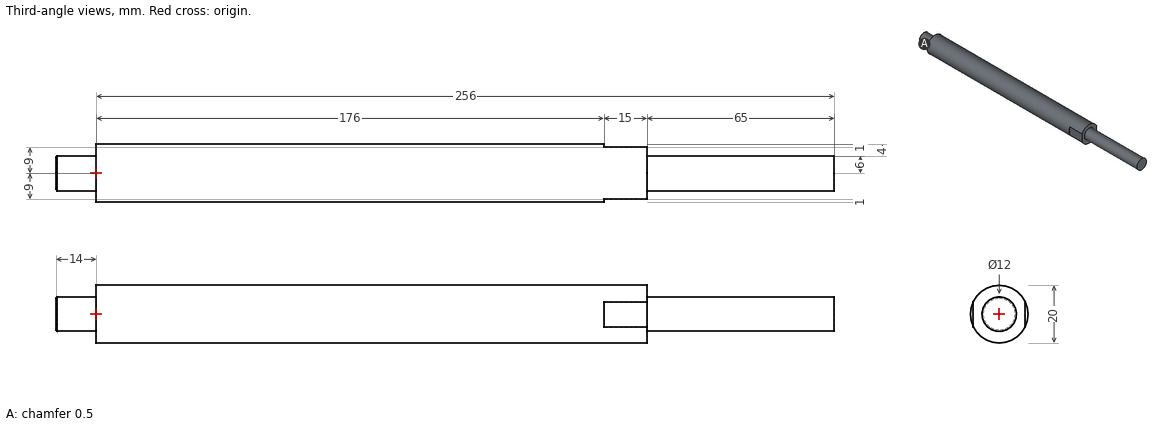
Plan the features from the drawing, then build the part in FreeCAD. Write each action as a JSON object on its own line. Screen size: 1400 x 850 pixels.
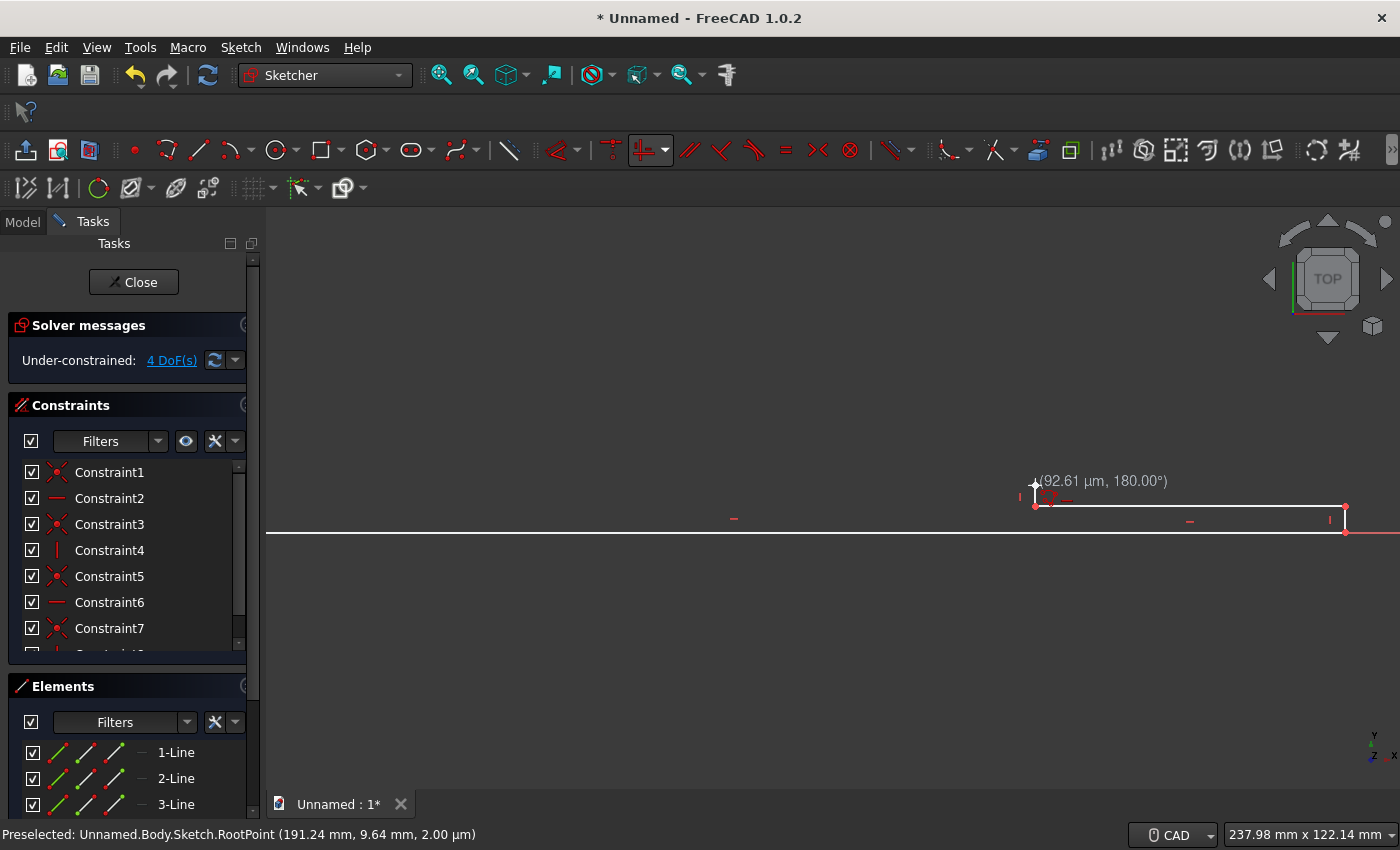
{"action": "scroll", "coordinate": [801, 485], "scroll_direction": "down", "scroll_amount": 3}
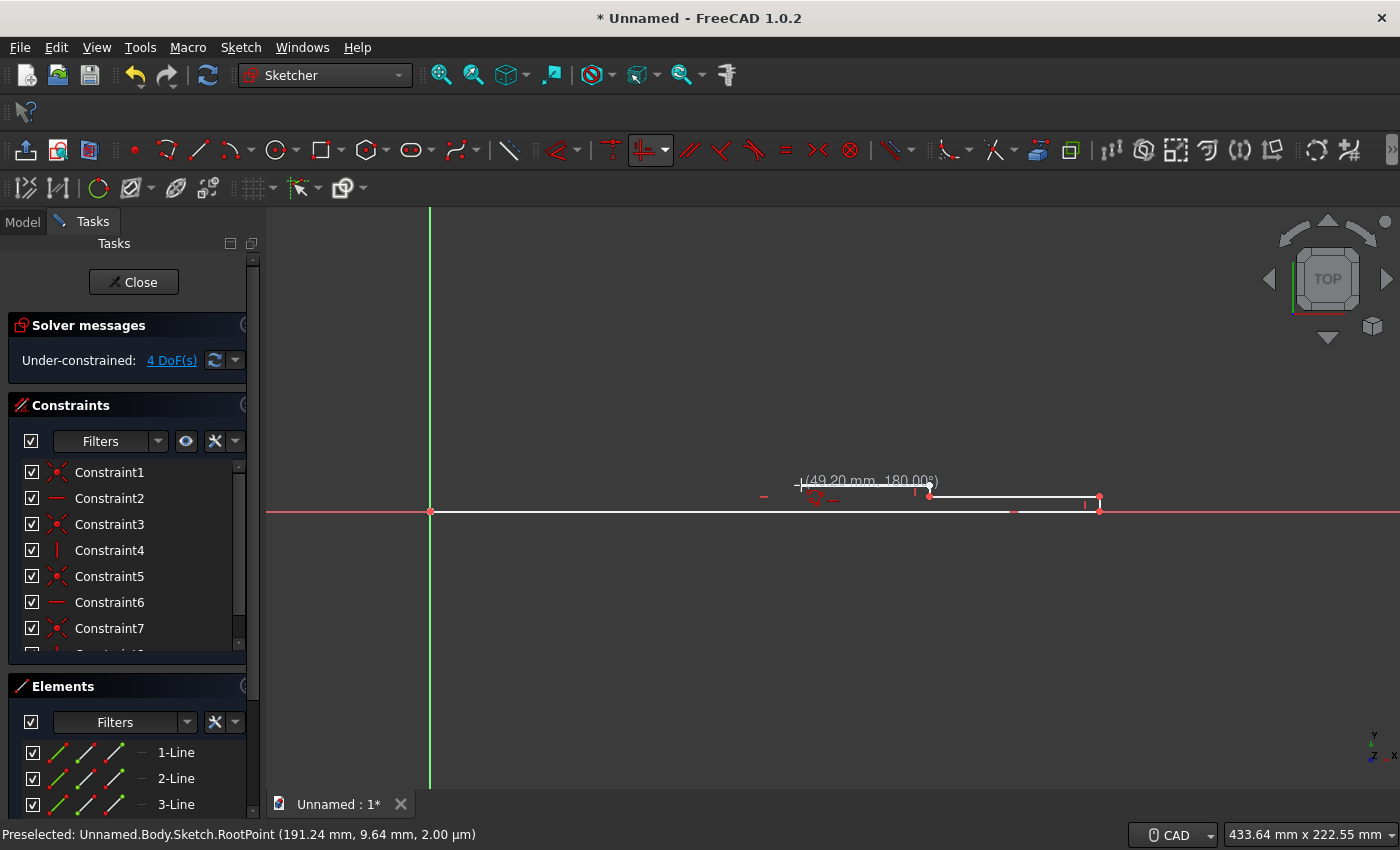
{"action": "left_click", "coordinate": [439, 485]}
{"action": "left_click", "coordinate": [430, 512]}
{"action": "key", "text": "Escape"}
{"action": "key", "text": "Escape"}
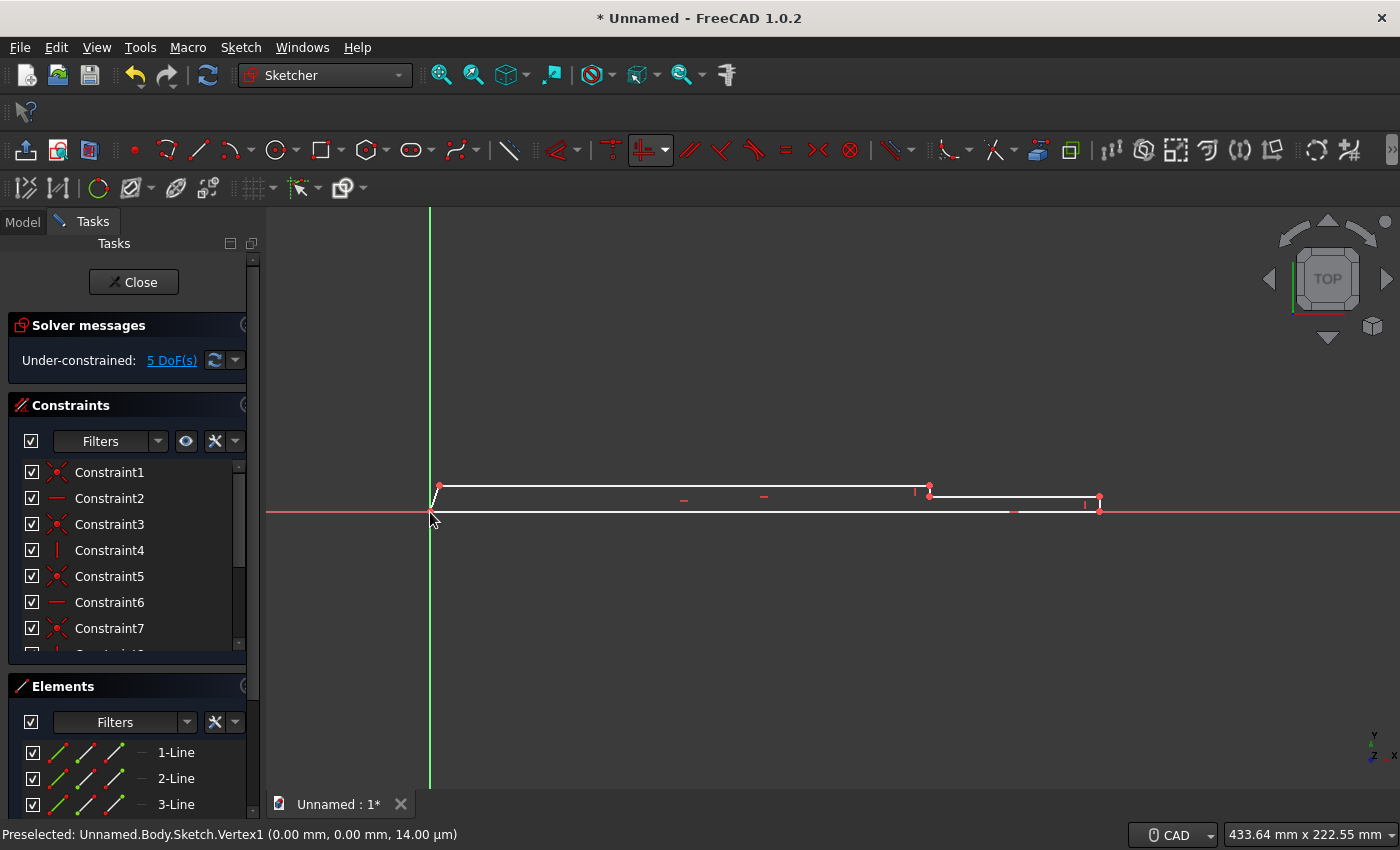
{"action": "scroll", "coordinate": [434, 501], "scroll_direction": "up", "scroll_amount": 2}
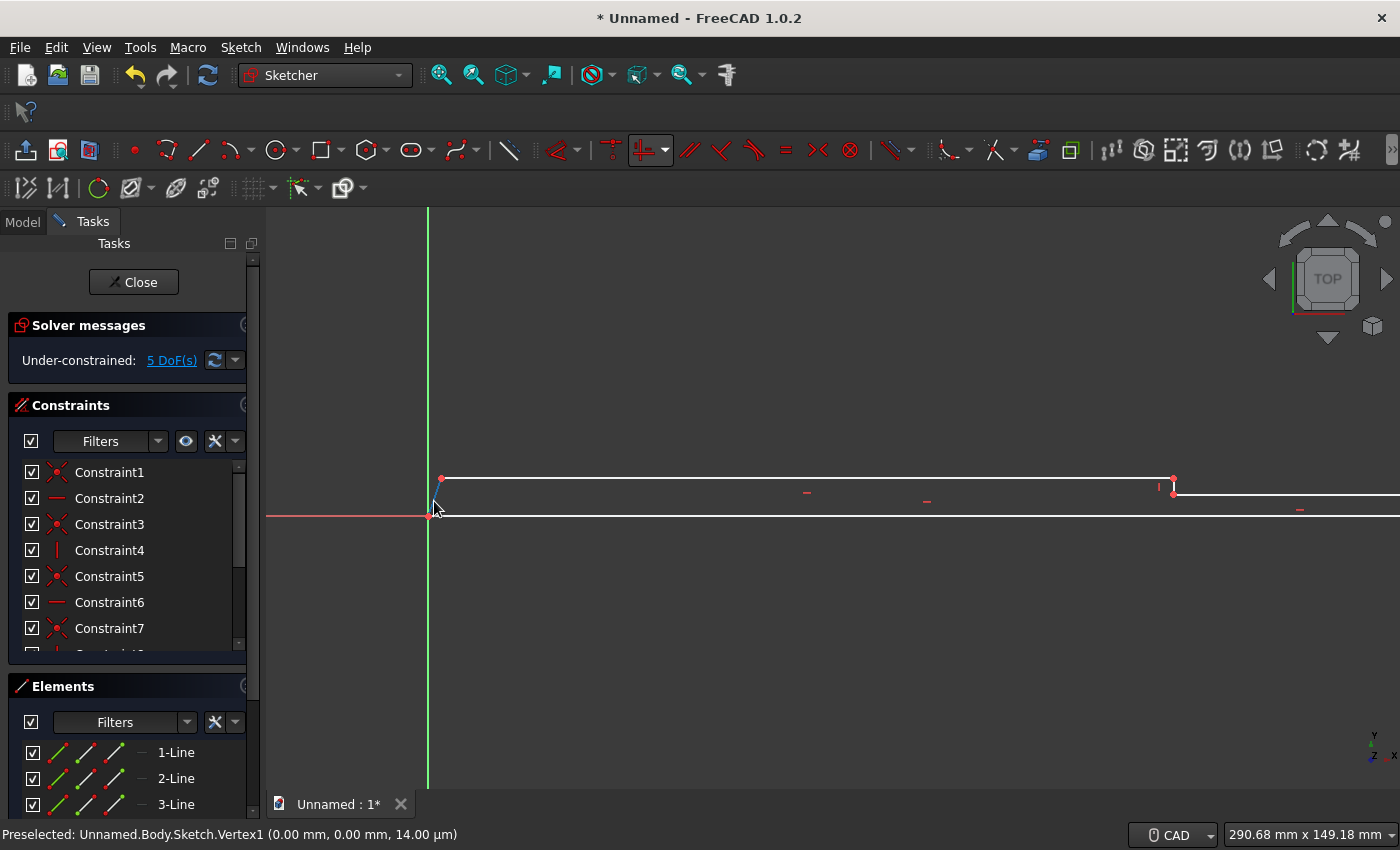
{"action": "left_click", "coordinate": [433, 501]}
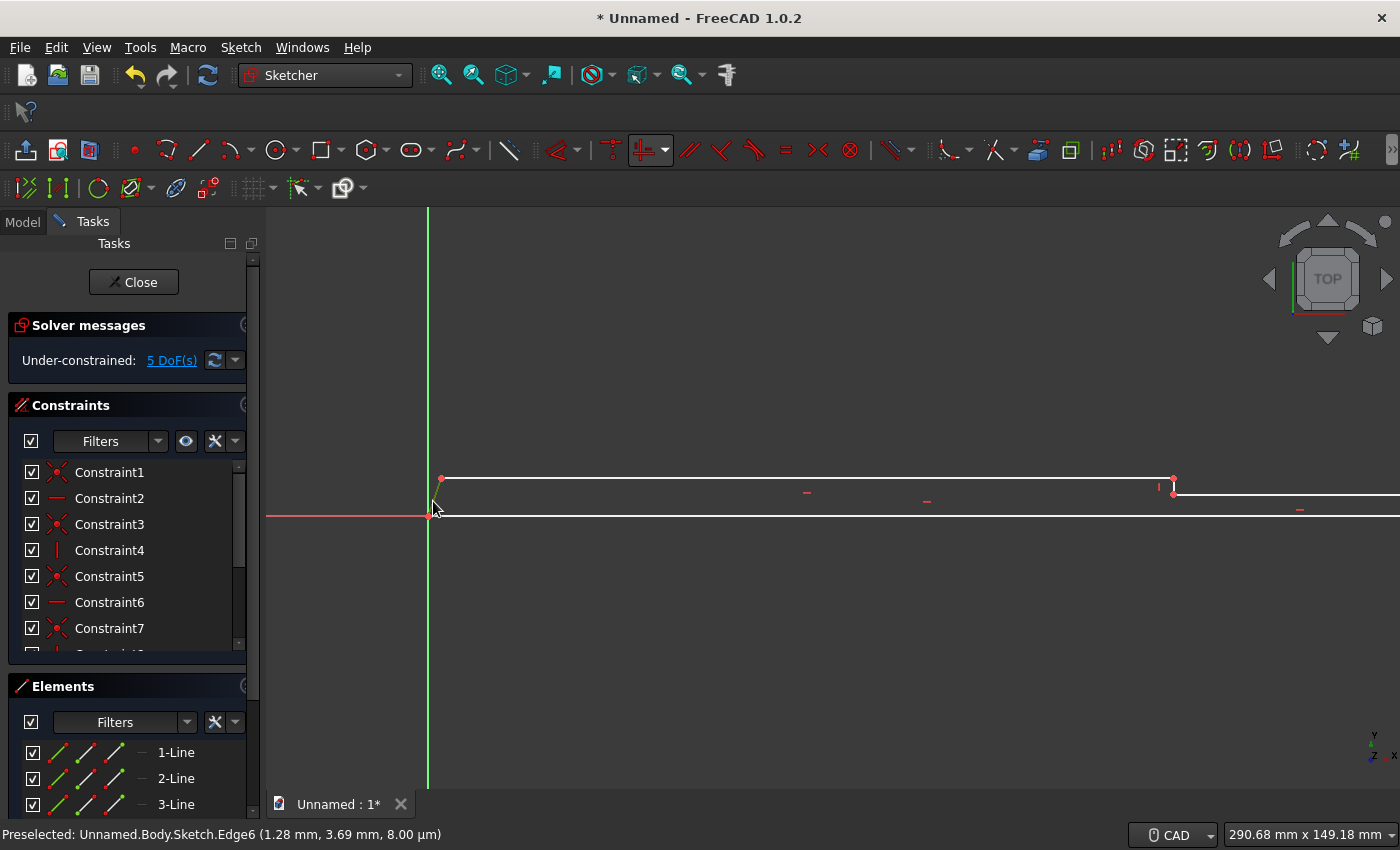
{"action": "key", "text": "v"}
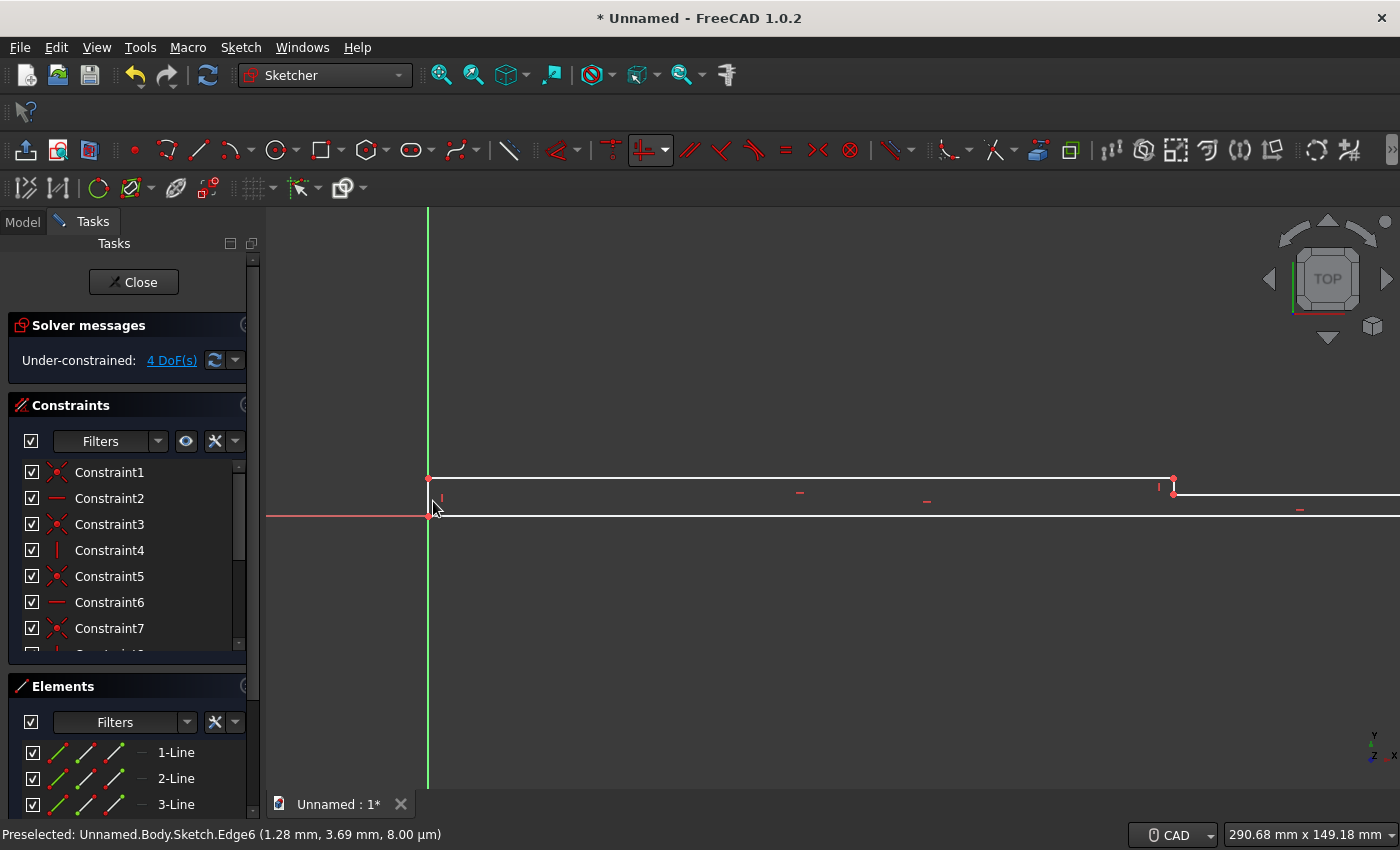
{"action": "key", "text": "d"}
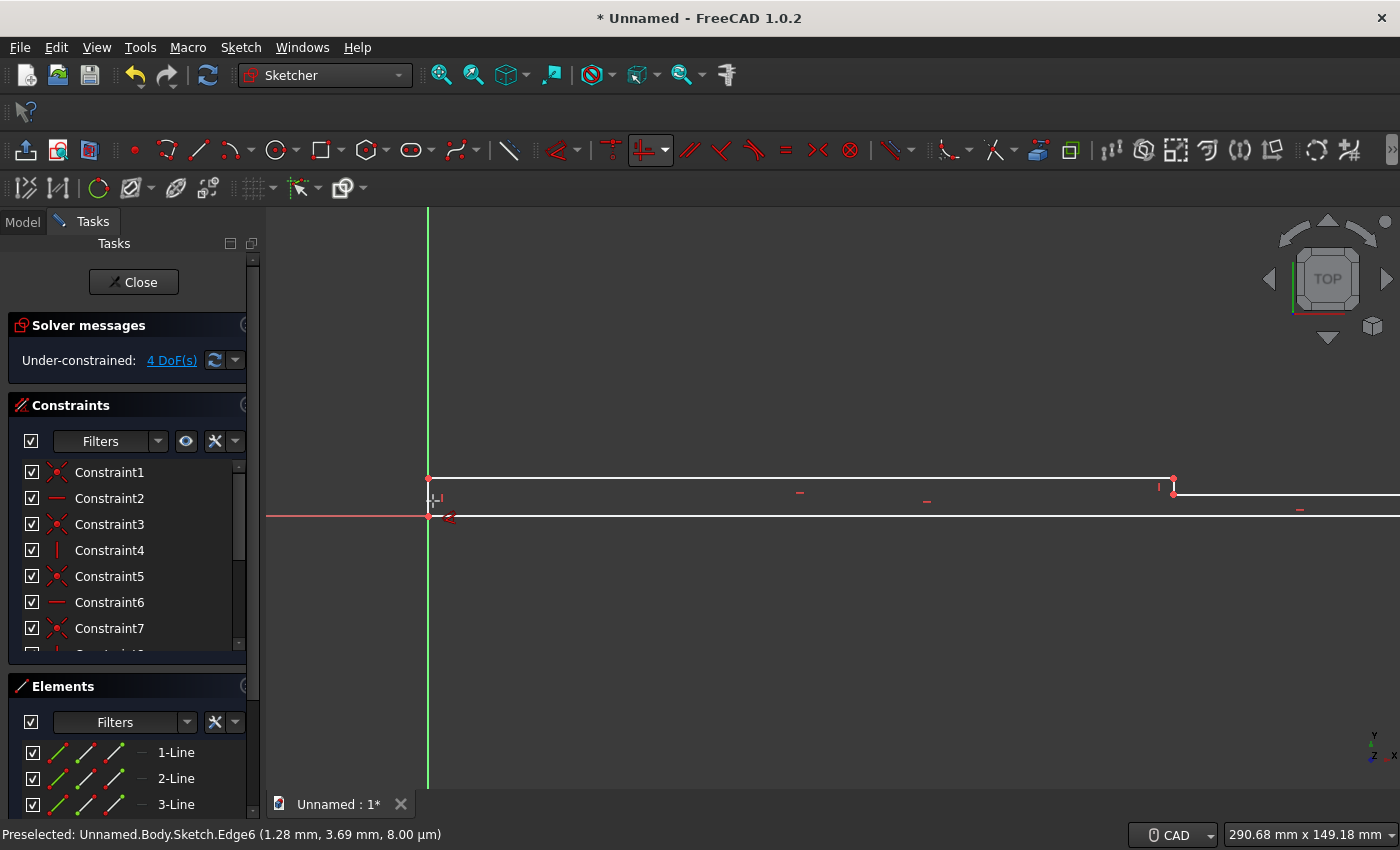
{"action": "scroll", "coordinate": [433, 500], "scroll_direction": "down", "scroll_amount": 2}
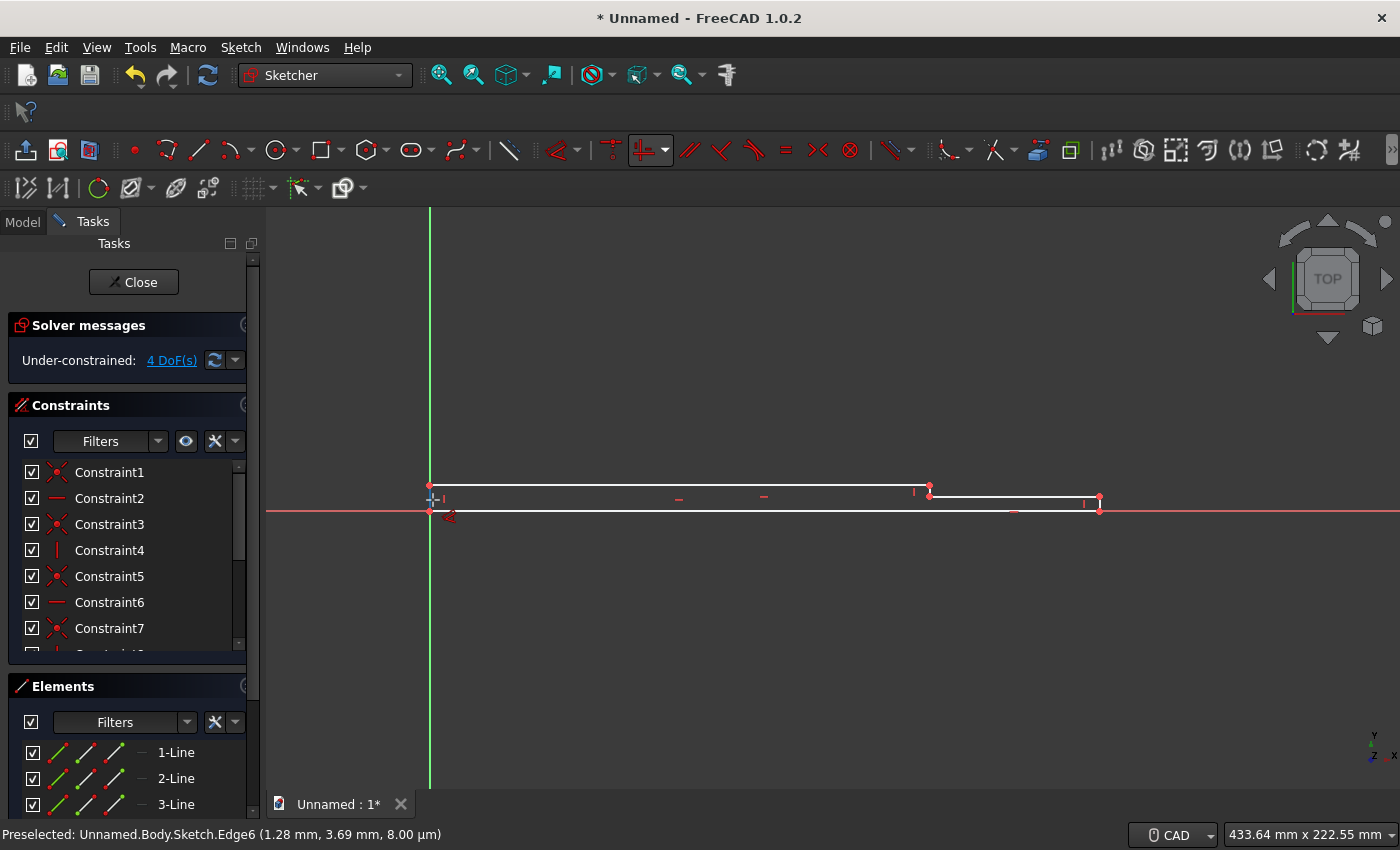
{"action": "scroll", "coordinate": [1100, 504], "scroll_direction": "up", "scroll_amount": 5}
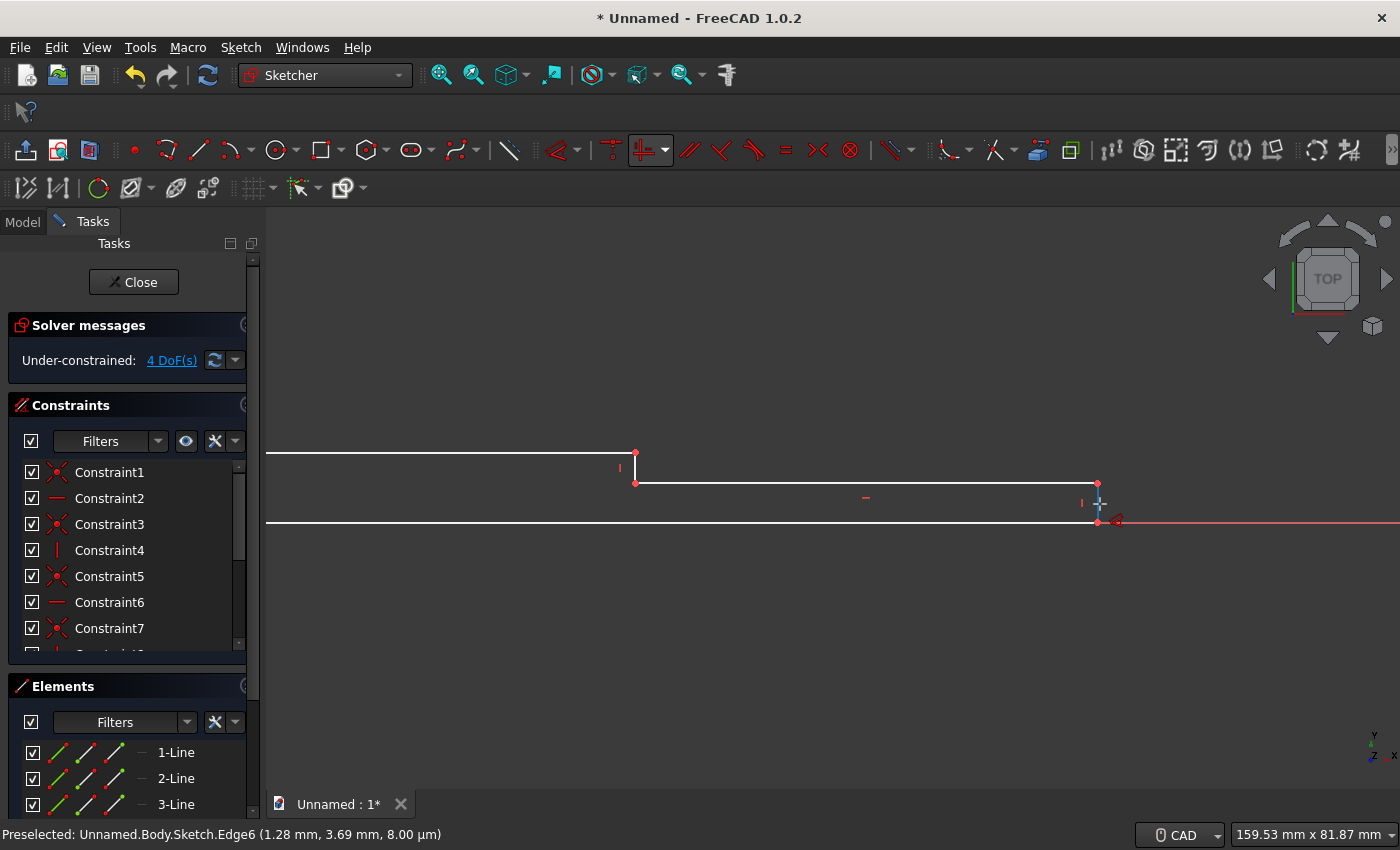
{"action": "left_click", "coordinate": [1098, 503]}
{"action": "left_click", "coordinate": [1132, 503]}